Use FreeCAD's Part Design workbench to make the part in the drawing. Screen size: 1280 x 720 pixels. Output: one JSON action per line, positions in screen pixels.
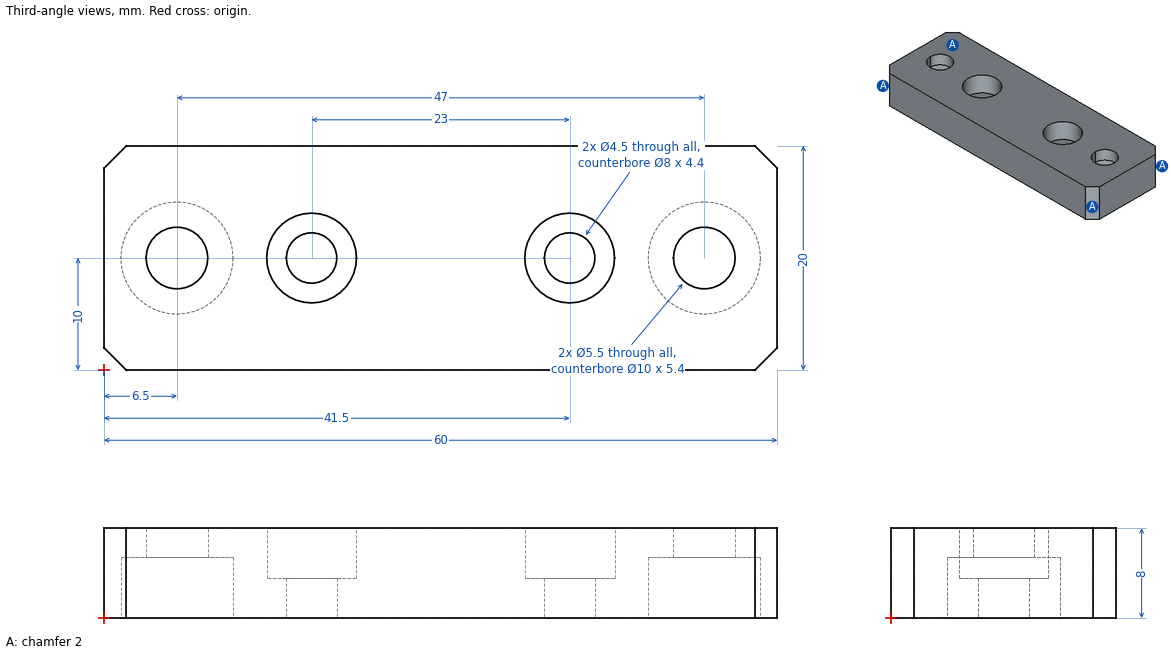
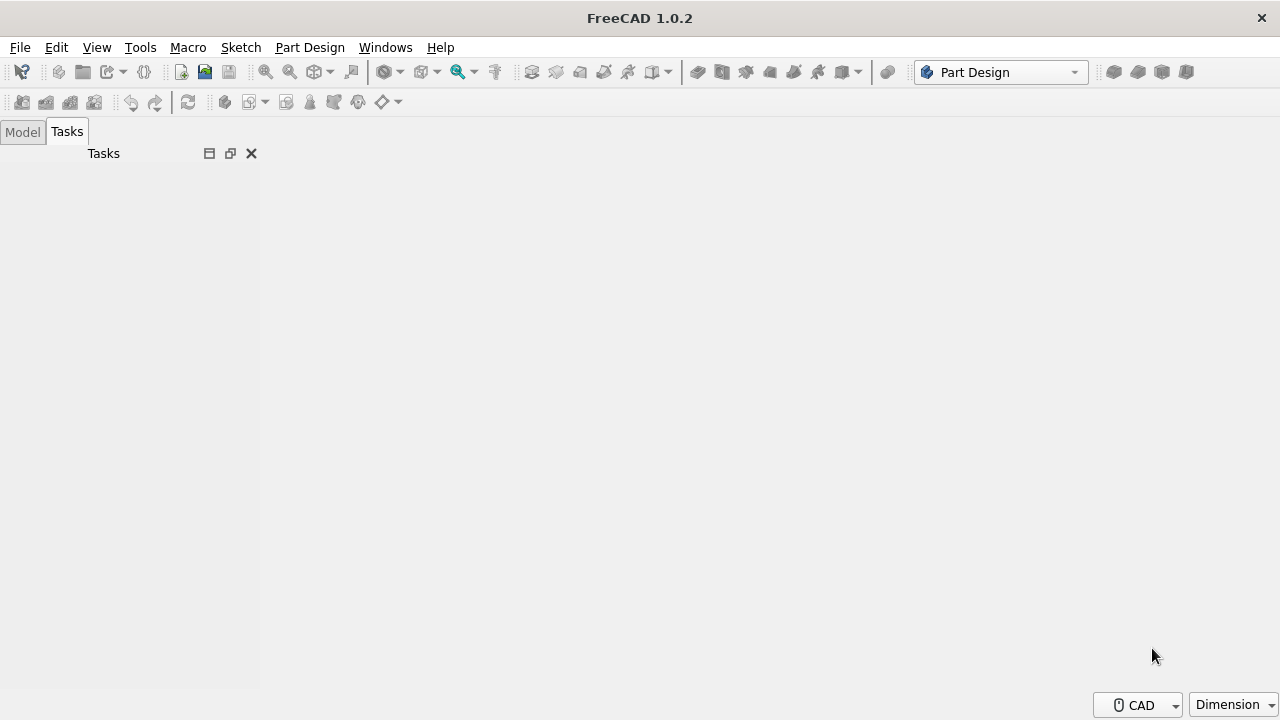
{"action": "key", "text": "ctrl+n"}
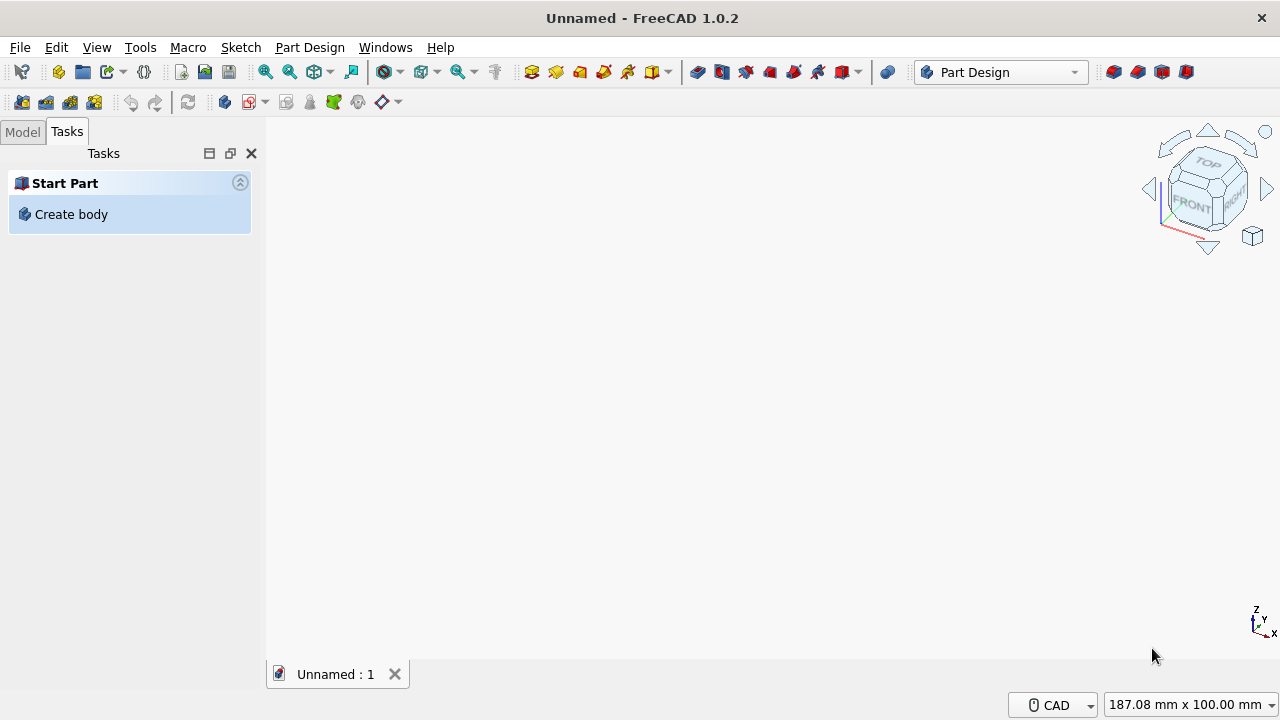
{"action": "left_click", "coordinate": [250, 102]}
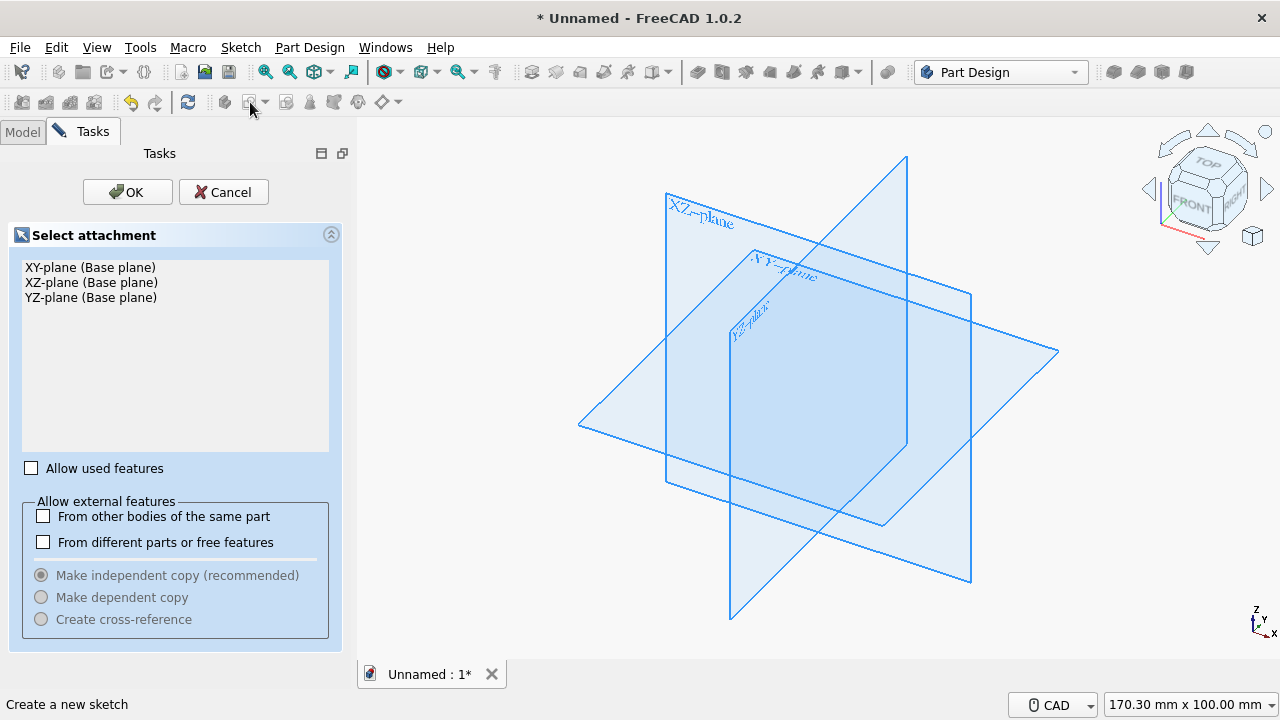
{"action": "left_click", "coordinate": [82, 268]}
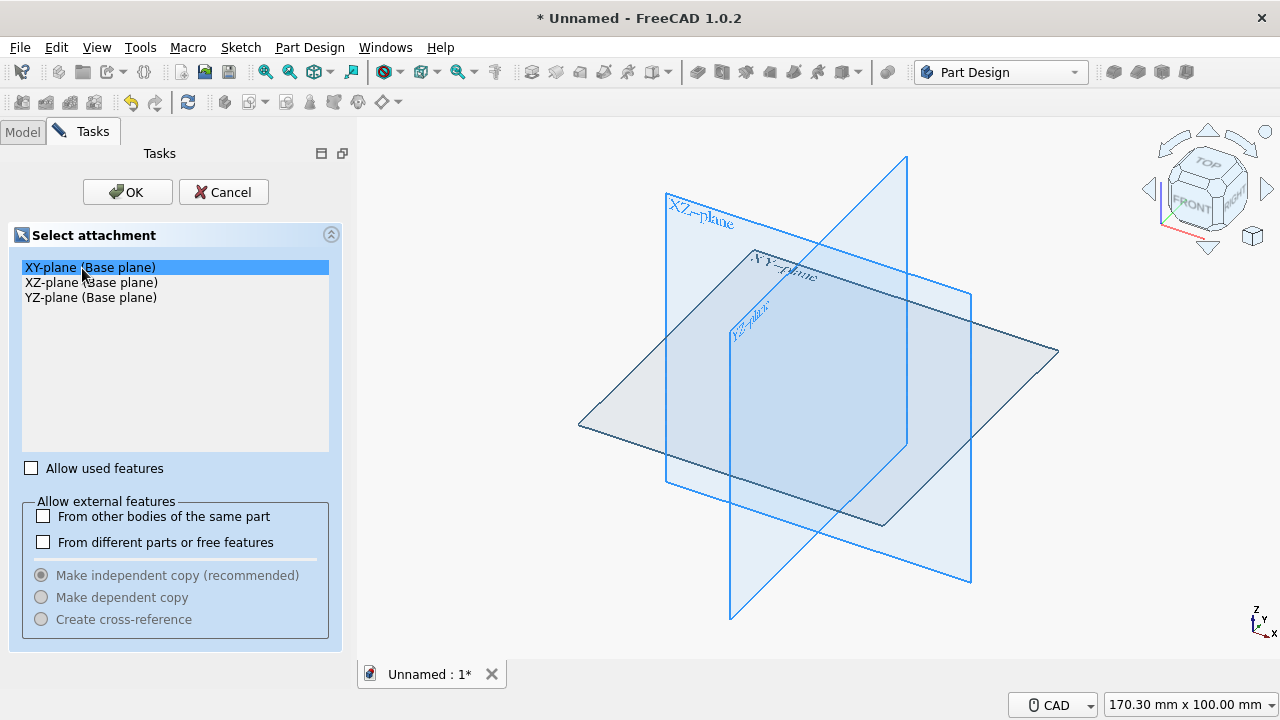
{"action": "left_click", "coordinate": [128, 192]}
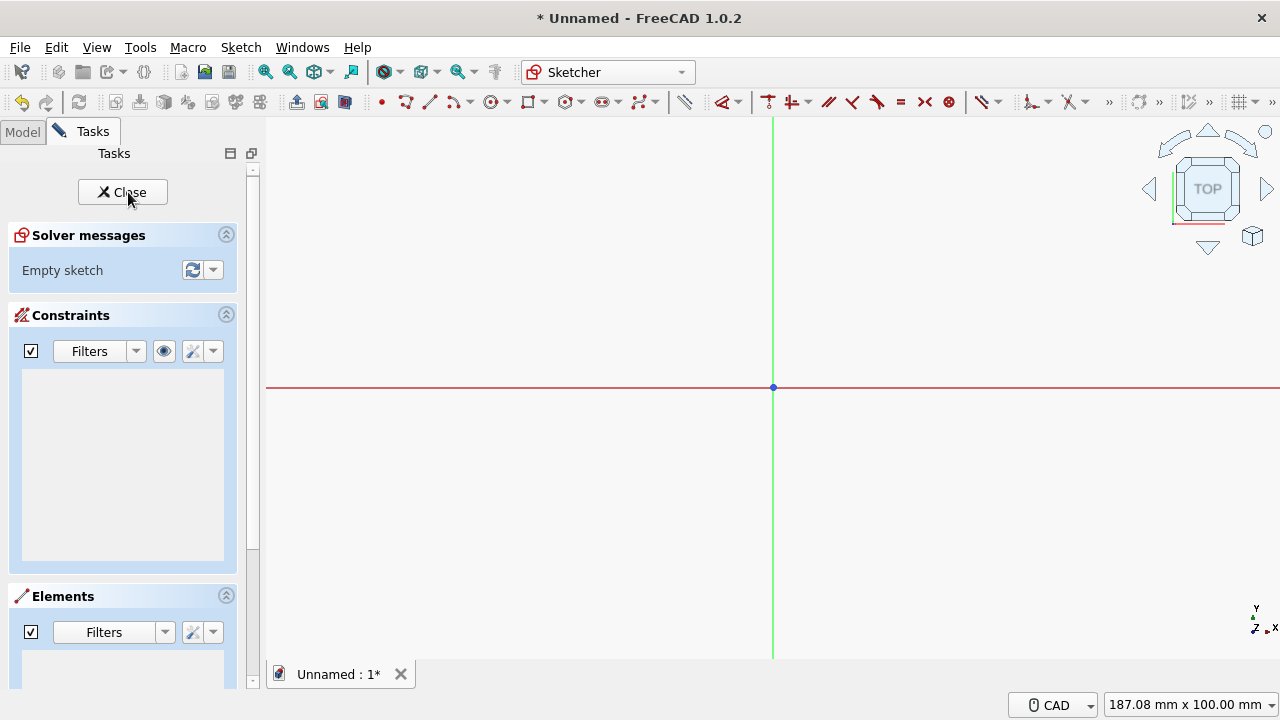
{"action": "scroll", "coordinate": [1115, 268], "scroll_direction": "up", "scroll_amount": 3}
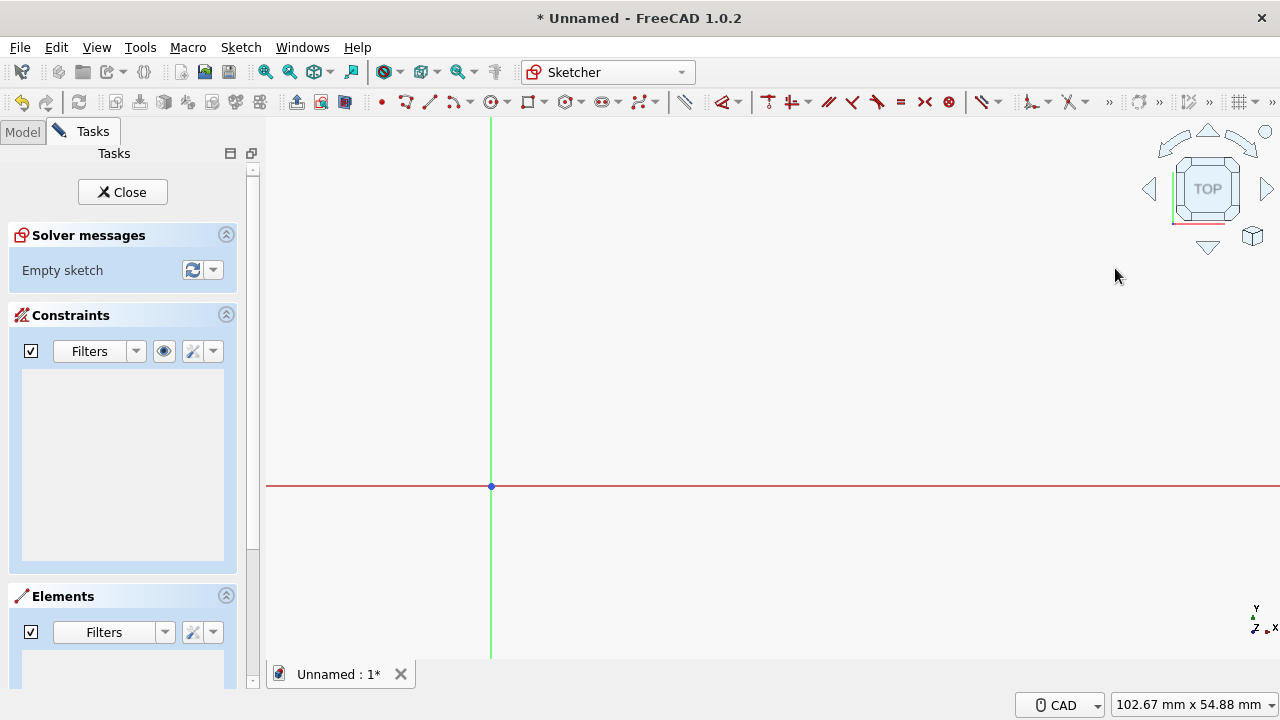
{"action": "key", "text": "g r"}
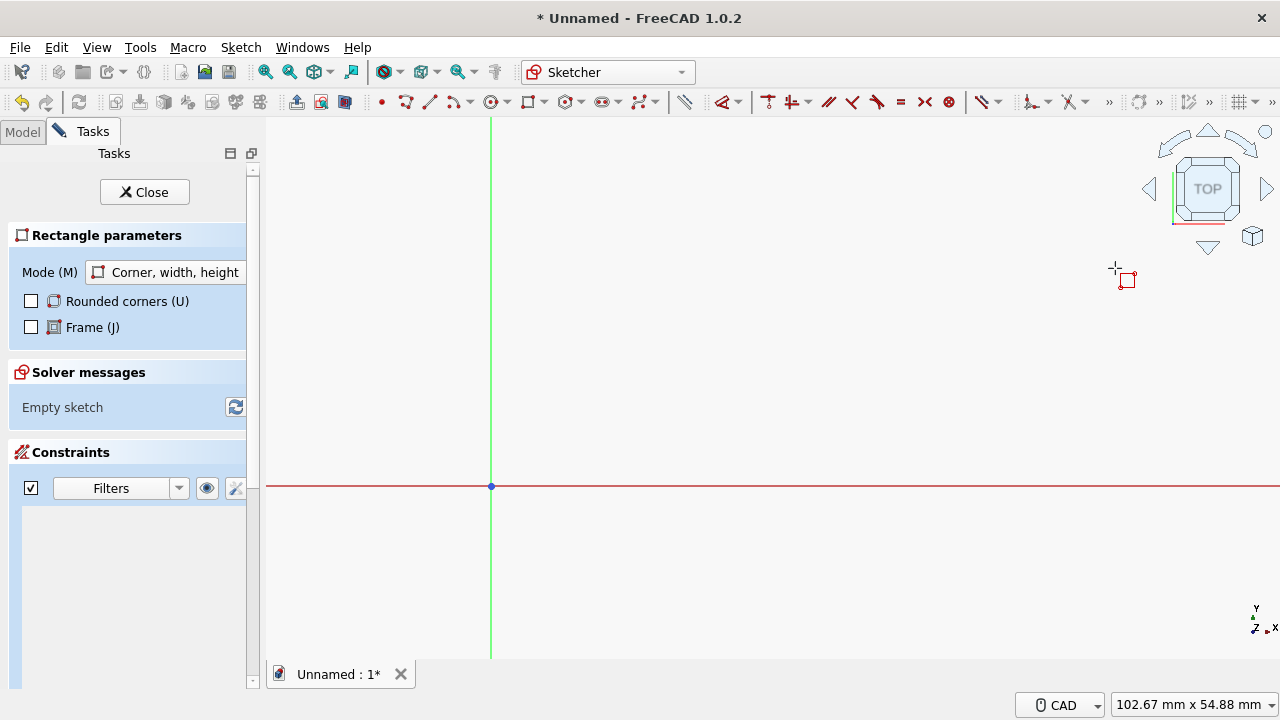
{"action": "left_click", "coordinate": [491, 486]}
{"action": "mouse_move", "coordinate": [1084, 289]}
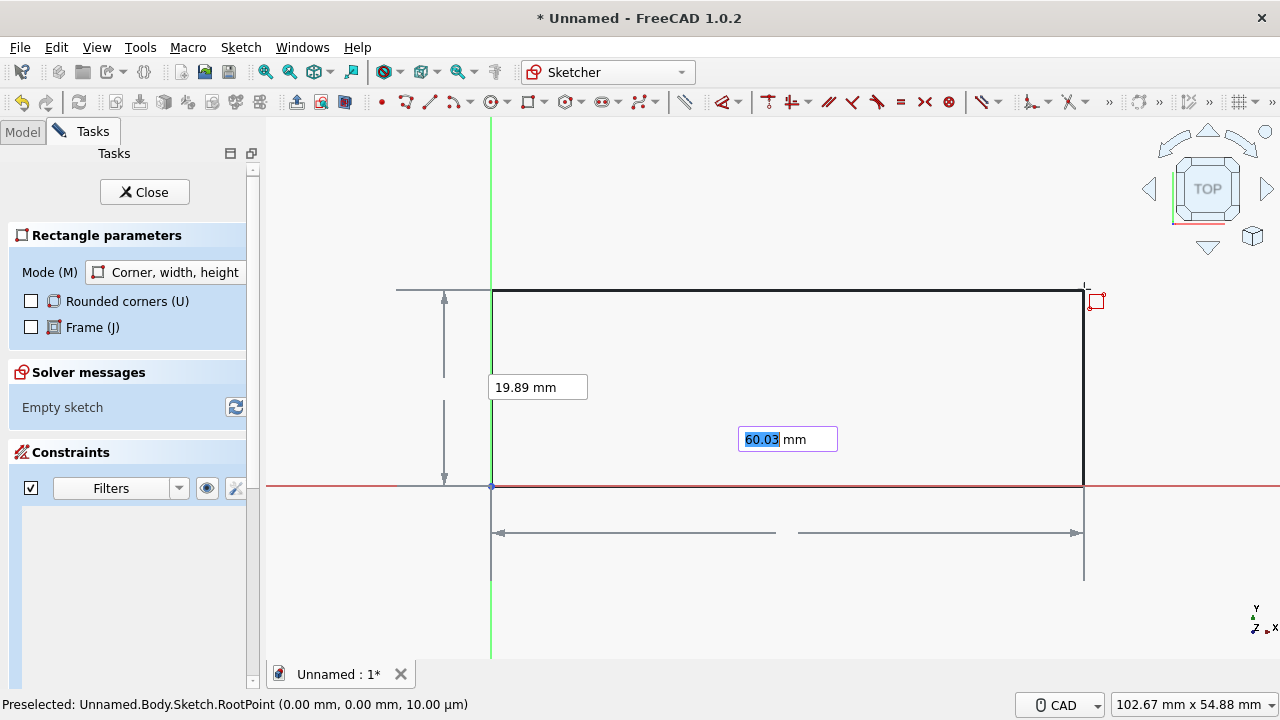
{"action": "type", "text": "60"}
{"action": "key", "text": "Tab"}
{"action": "type", "text": "20"}
{"action": "key", "text": "Return"}
{"action": "key", "text": "Escape"}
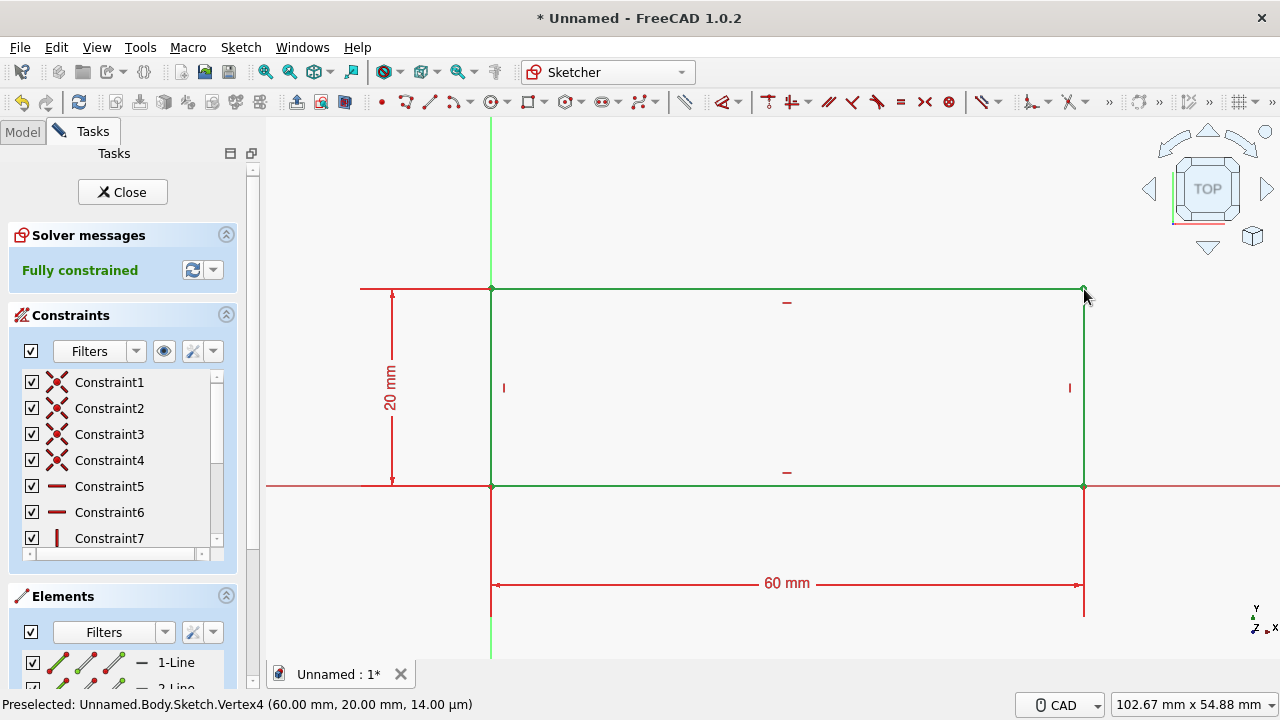
{"action": "left_click", "coordinate": [123, 192]}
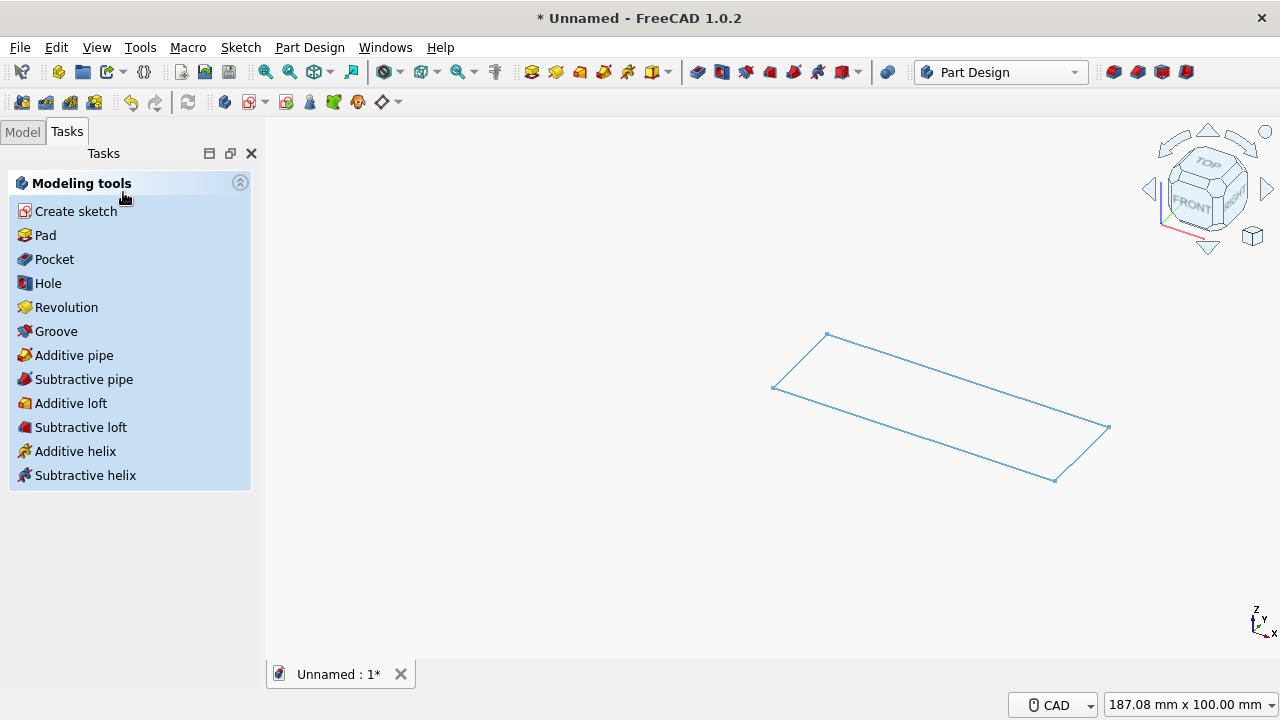
{"action": "left_click", "coordinate": [532, 72]}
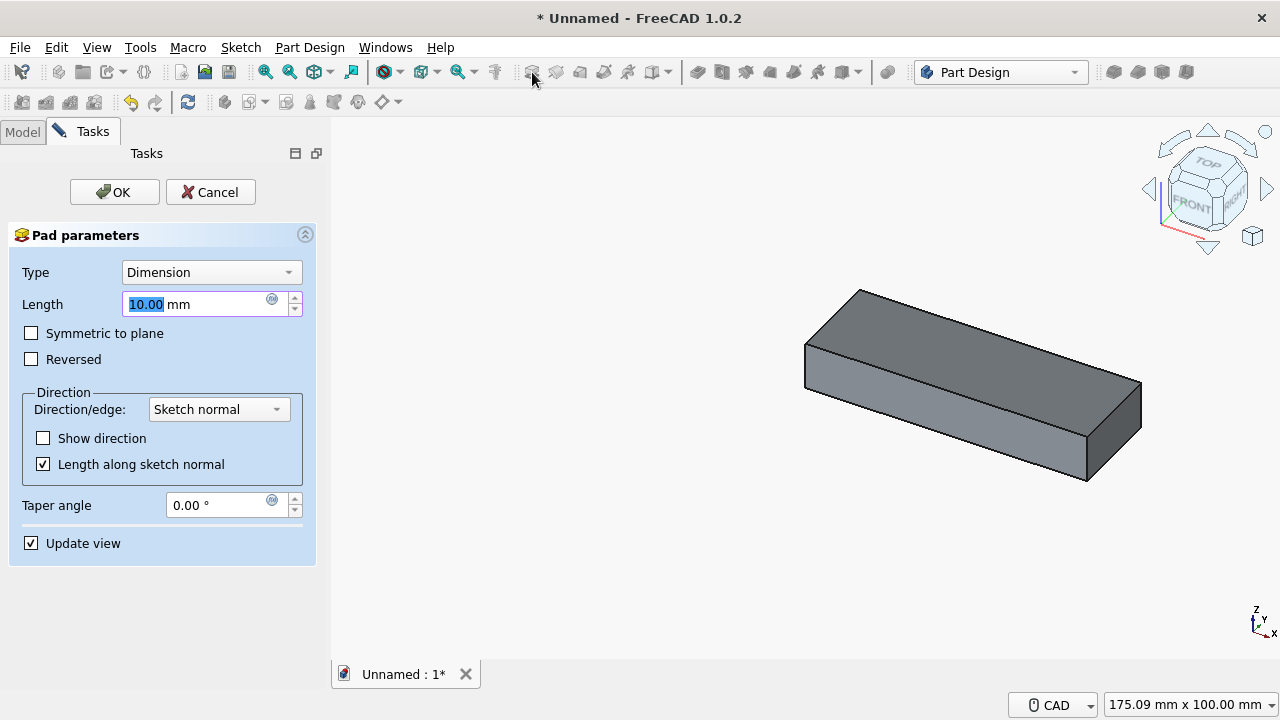
{"action": "type", "text": "8"}
{"action": "key", "text": "Tab"}